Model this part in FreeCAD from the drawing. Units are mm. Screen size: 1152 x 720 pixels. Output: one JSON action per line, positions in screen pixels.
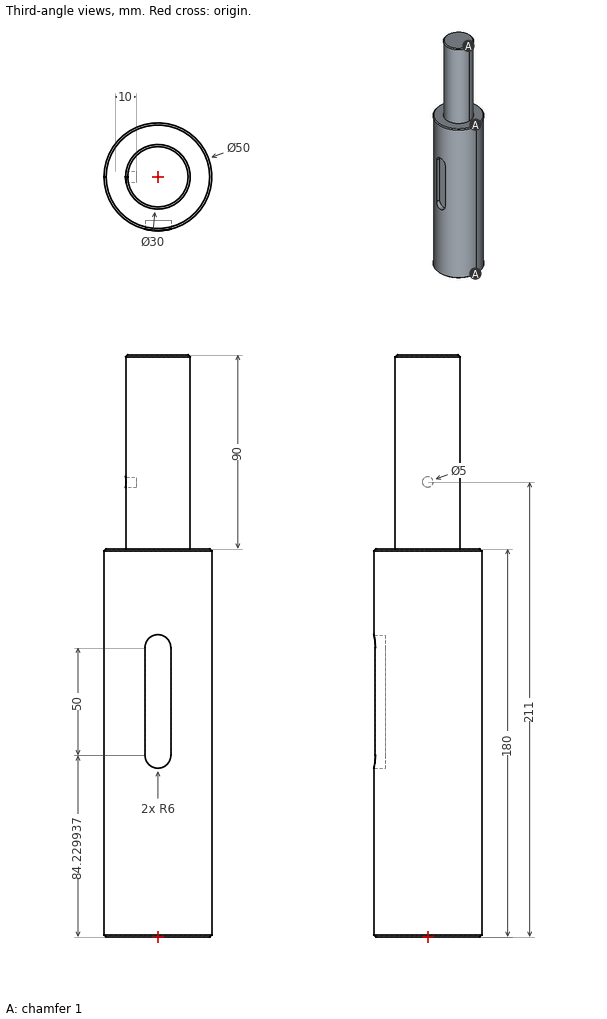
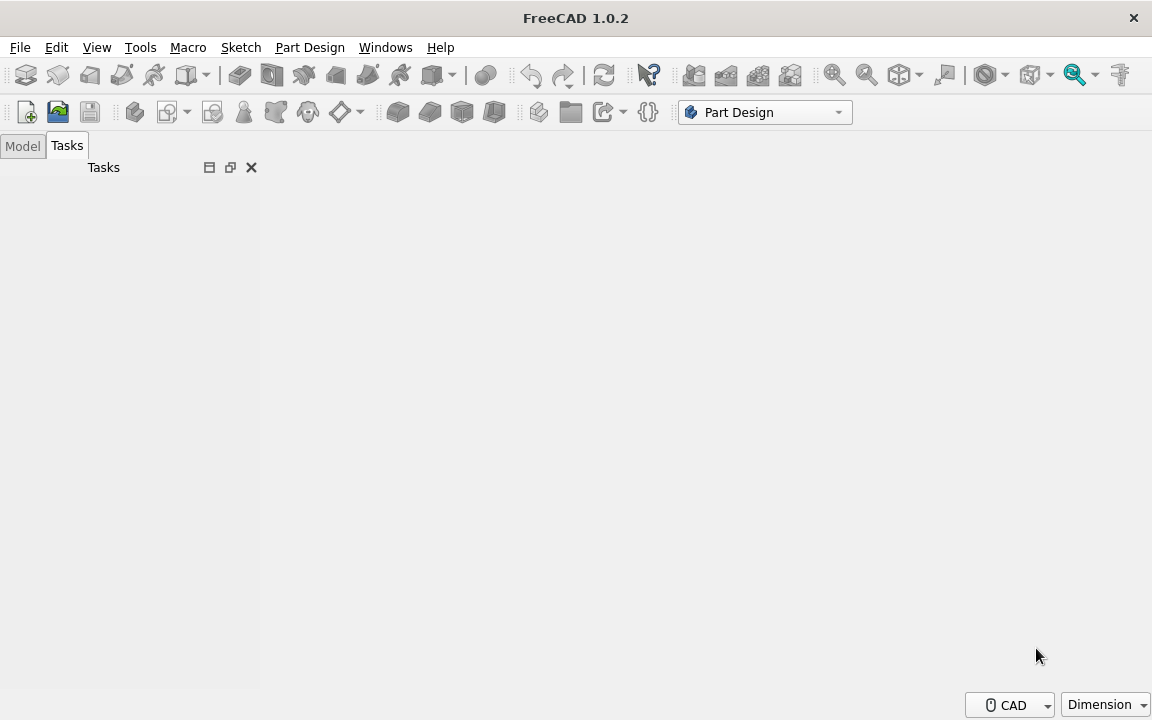
{"action": "key", "text": "ctrl+n"}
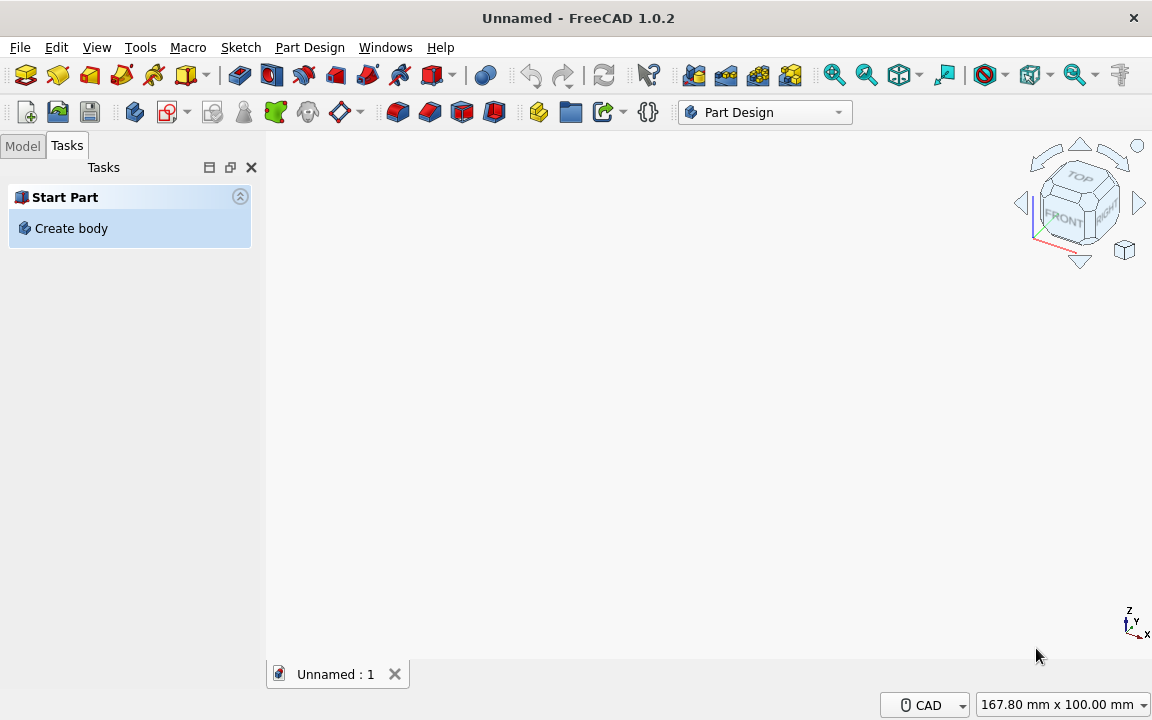
{"action": "left_click", "coordinate": [168, 112]}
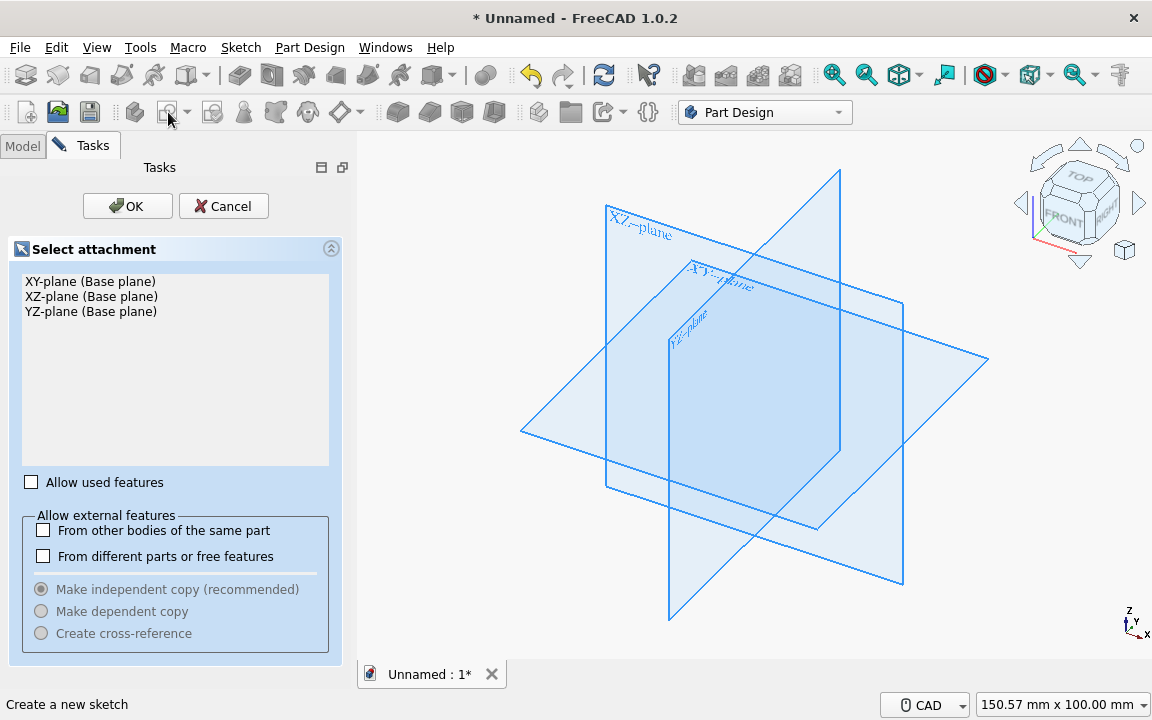
{"action": "left_click", "coordinate": [82, 282]}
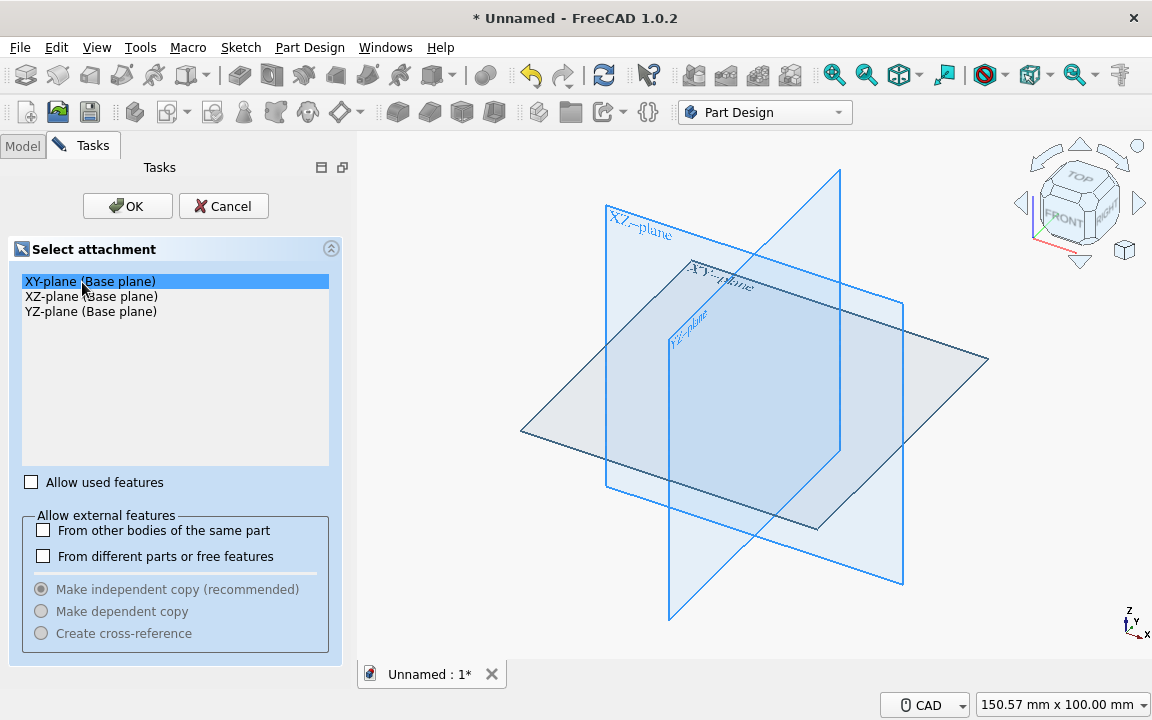
{"action": "left_click", "coordinate": [128, 206]}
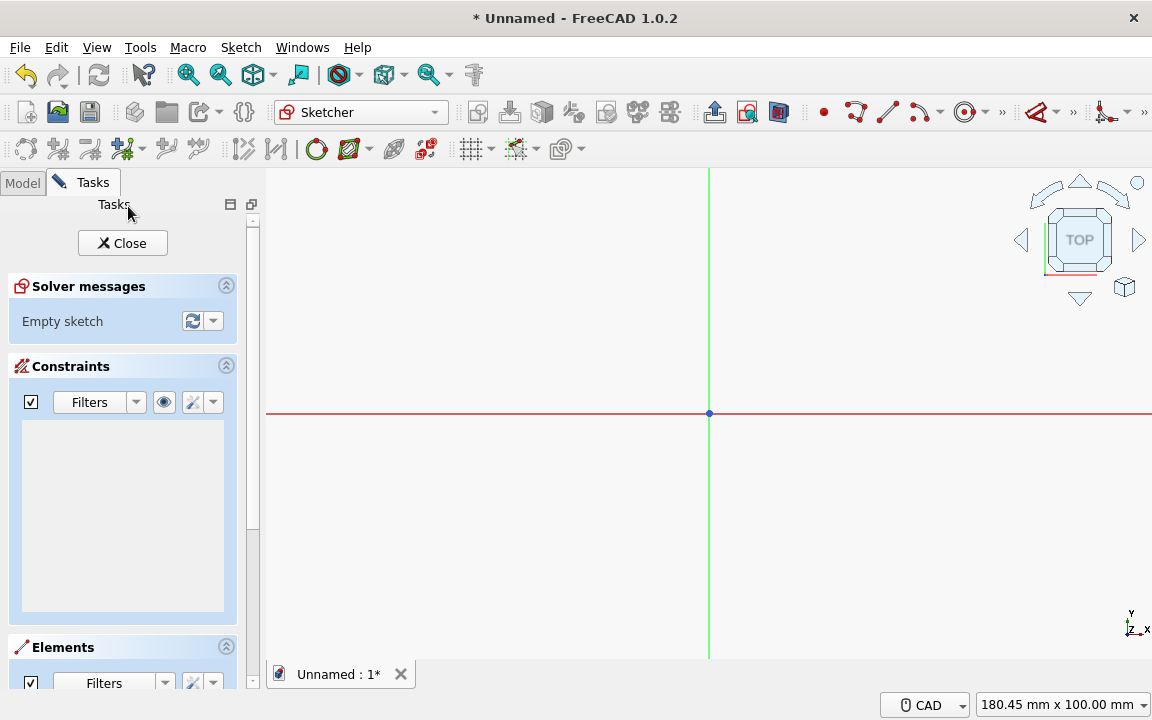
{"action": "key", "text": "g c"}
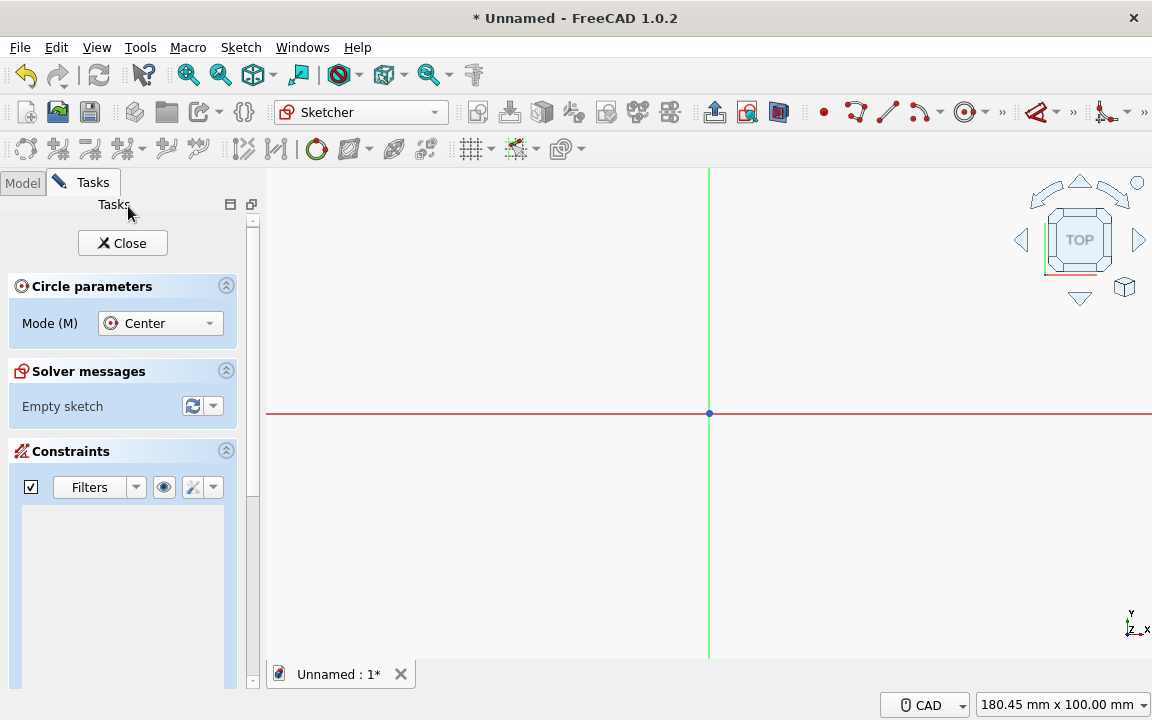
{"action": "left_click", "coordinate": [709, 414]}
{"action": "left_click", "coordinate": [796, 327]}
{"action": "key", "text": "Escape"}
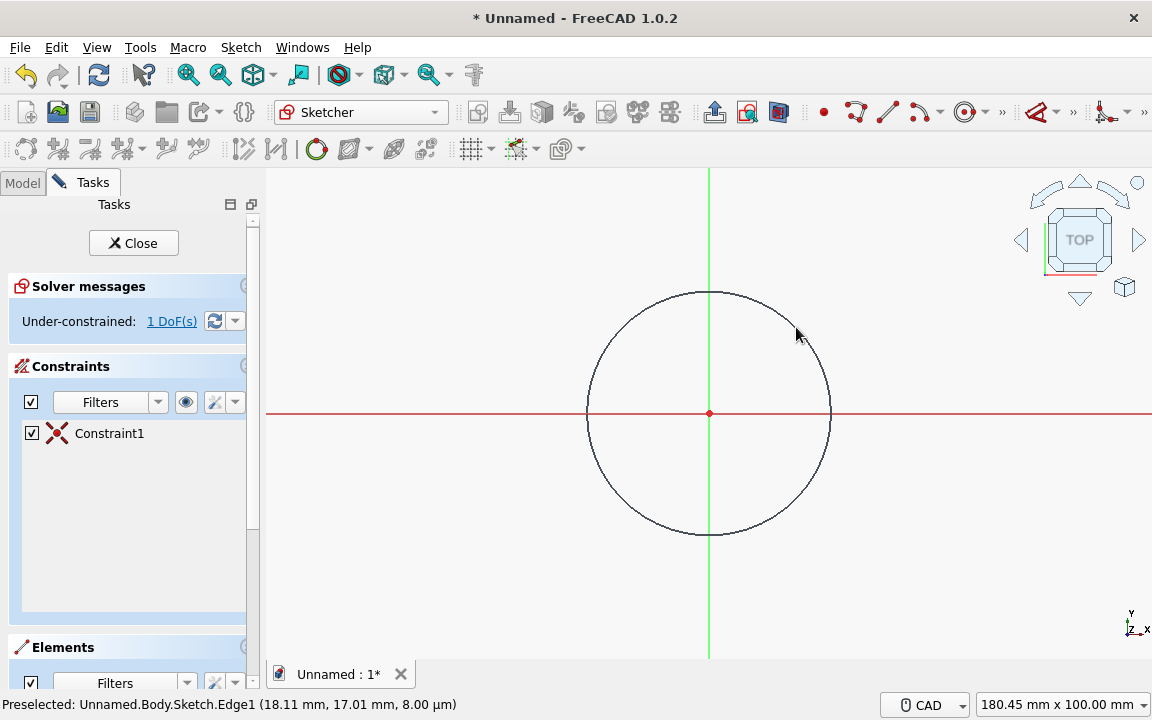
{"action": "key", "text": "d"}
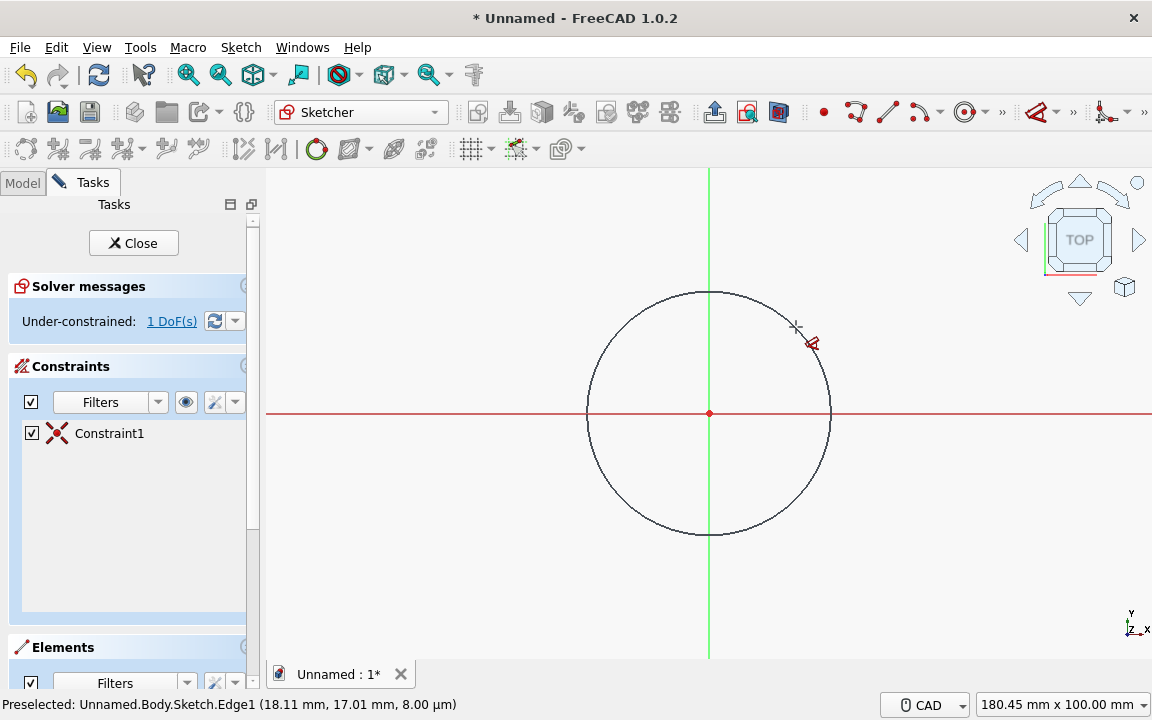
{"action": "left_click", "coordinate": [795, 327]}
{"action": "left_click", "coordinate": [818, 304]}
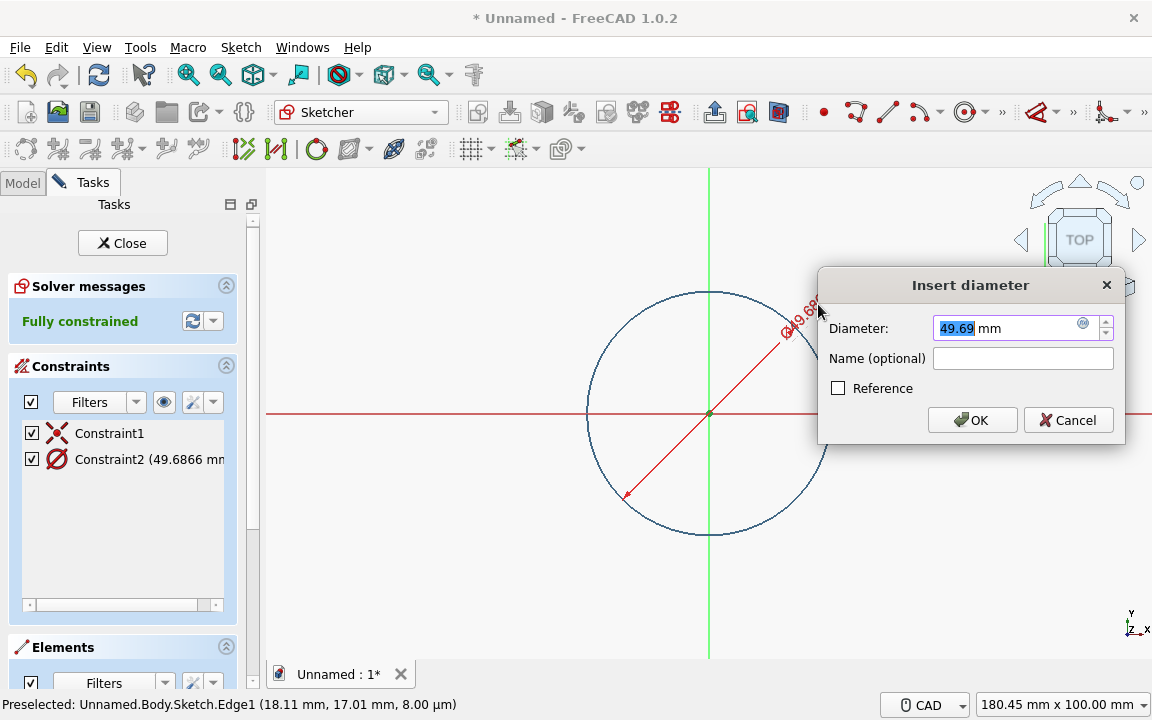
{"action": "type", "text": "50"}
{"action": "key", "text": "Return"}
{"action": "key", "text": "Escape"}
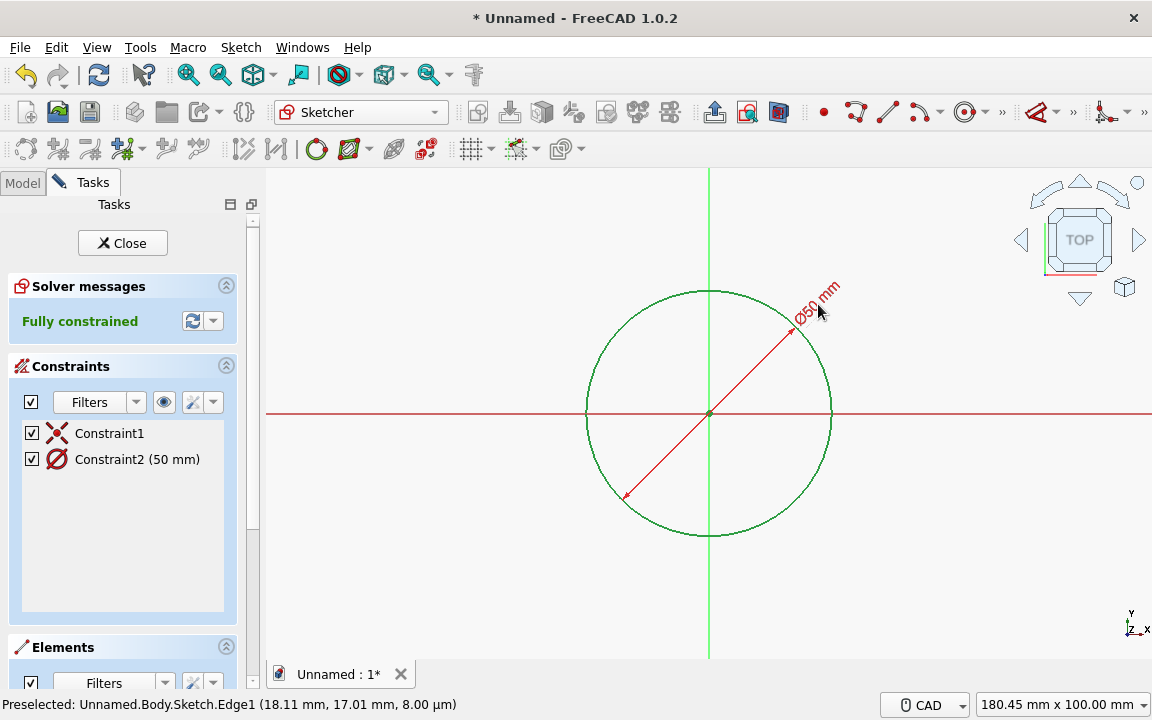
{"action": "left_click", "coordinate": [123, 243]}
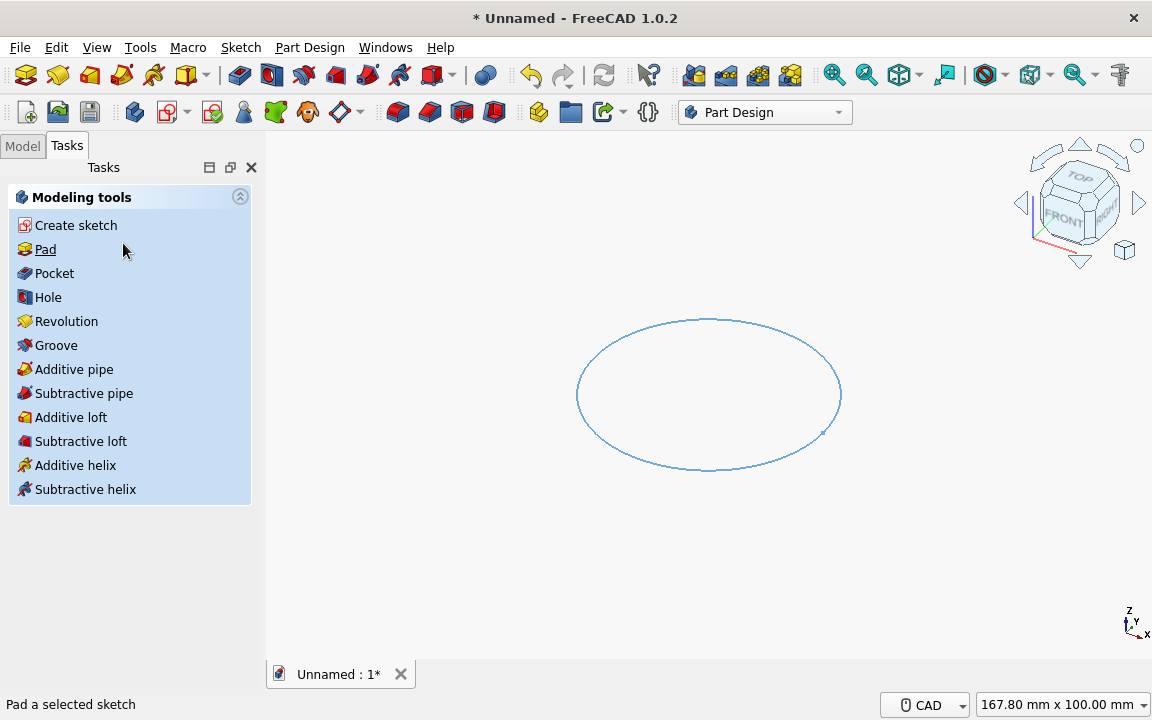
{"action": "left_click", "coordinate": [26, 76]}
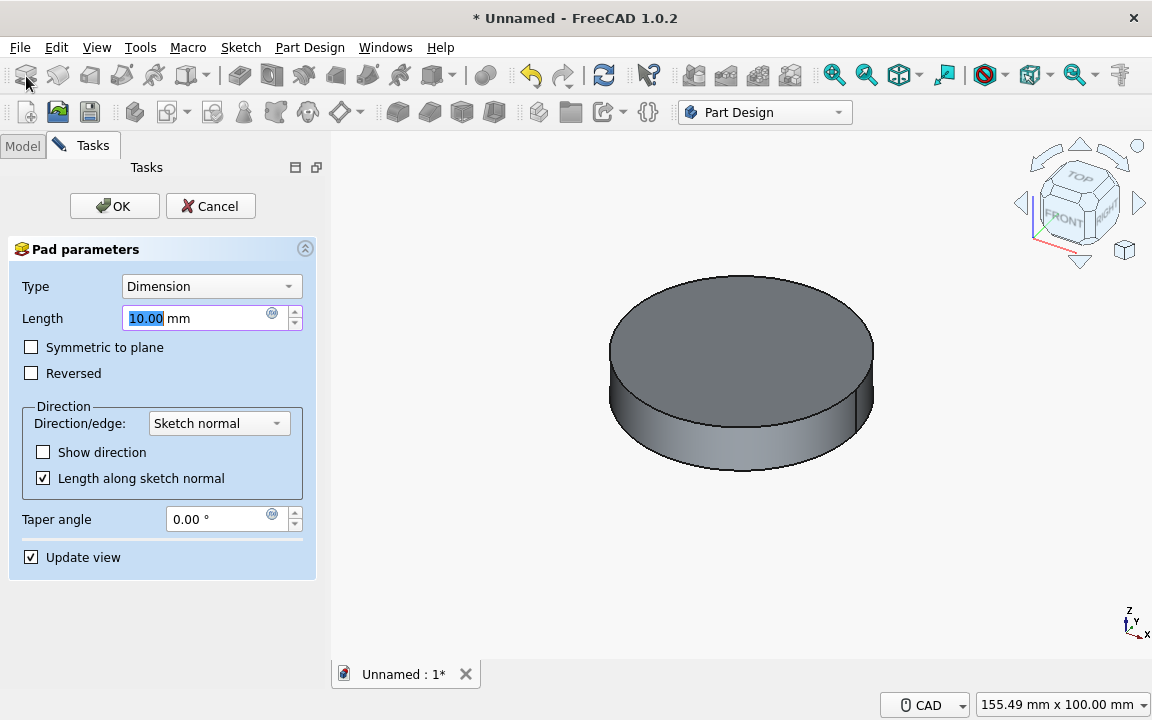
{"action": "type", "text": "180"}
{"action": "key", "text": "Tab"}